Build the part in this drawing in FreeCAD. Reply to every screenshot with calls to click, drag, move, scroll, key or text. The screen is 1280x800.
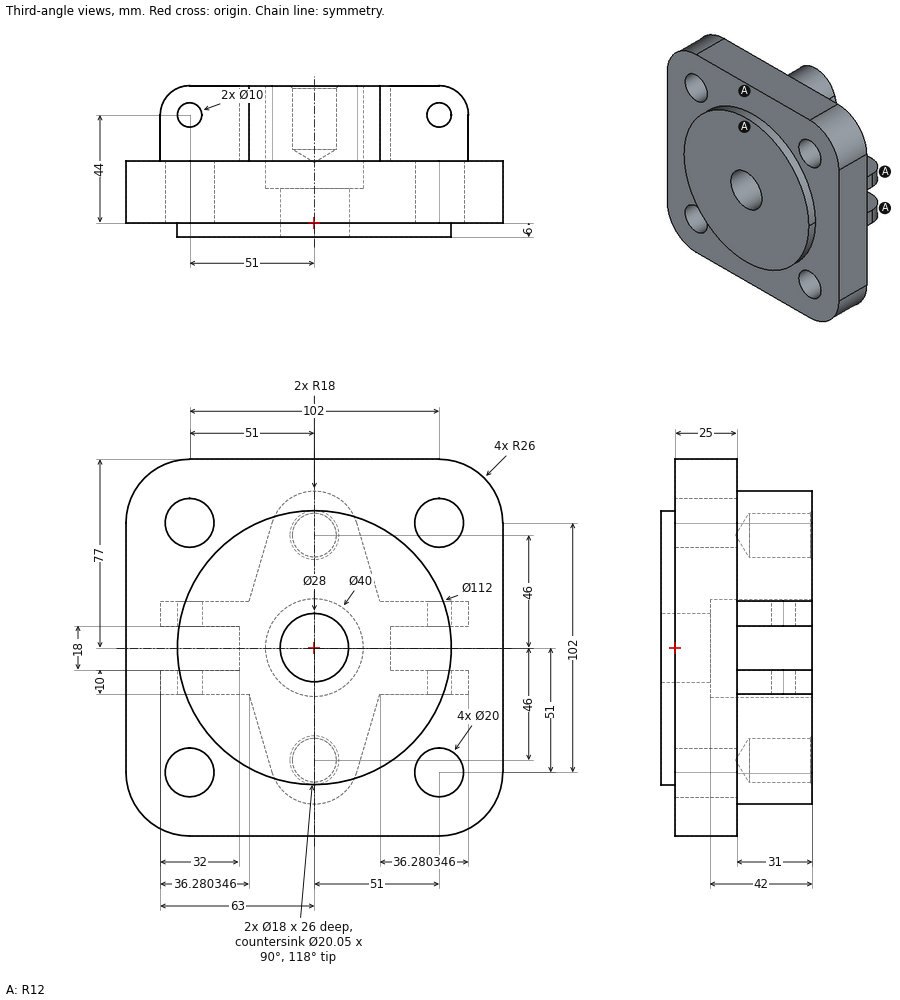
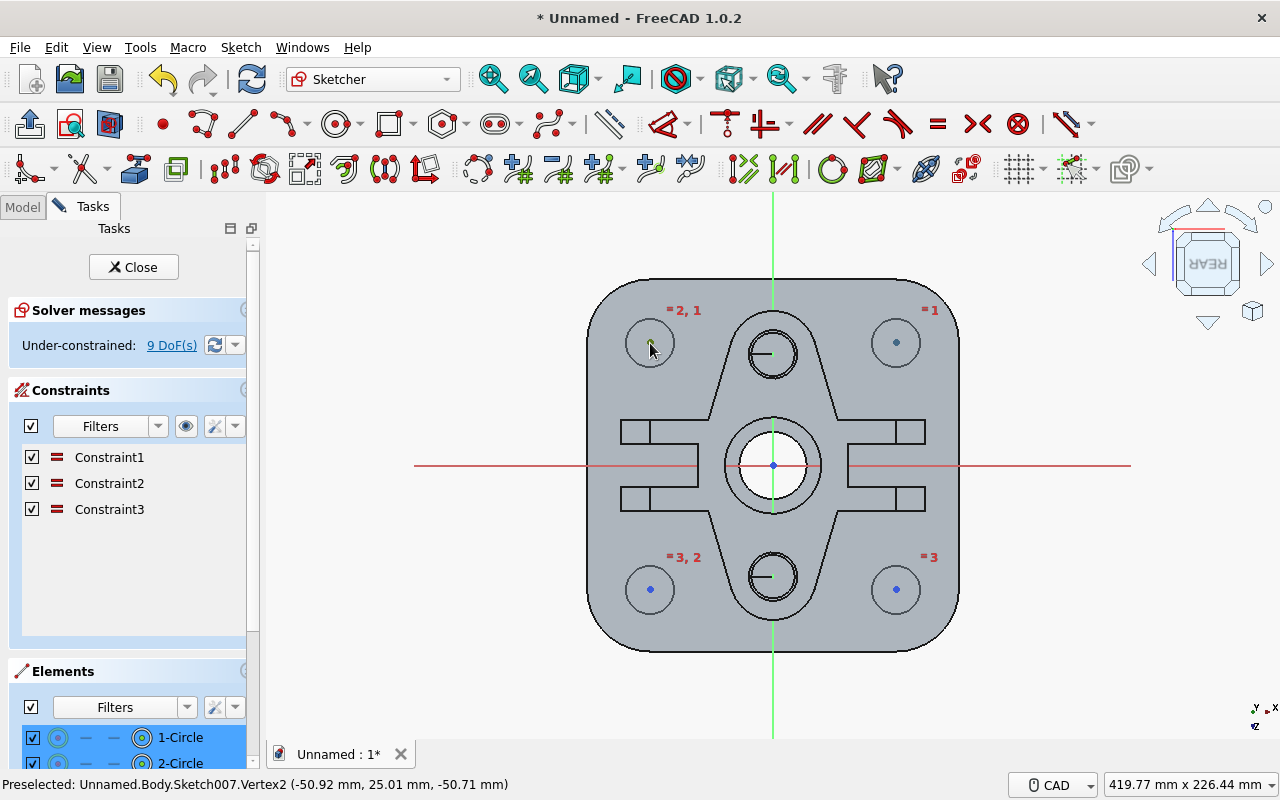
click(773, 676)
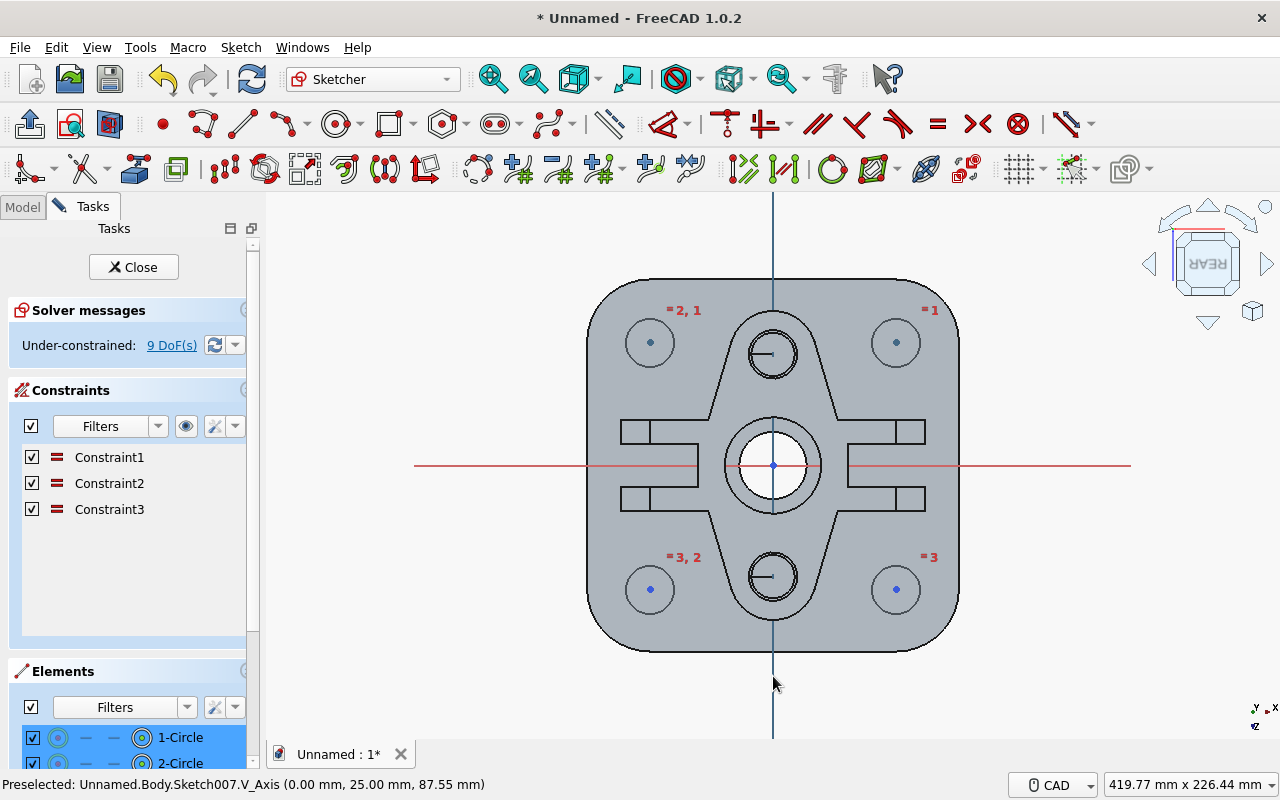
key(s)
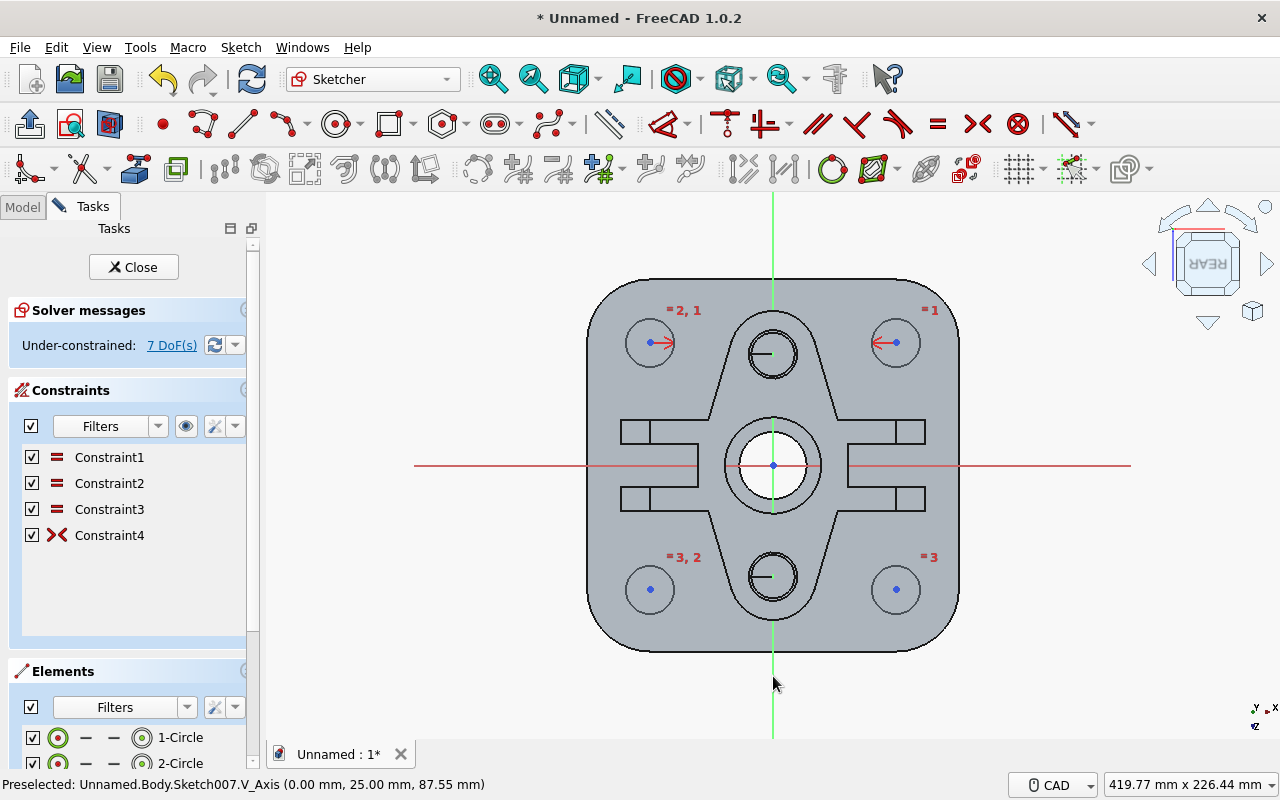
click(650, 343)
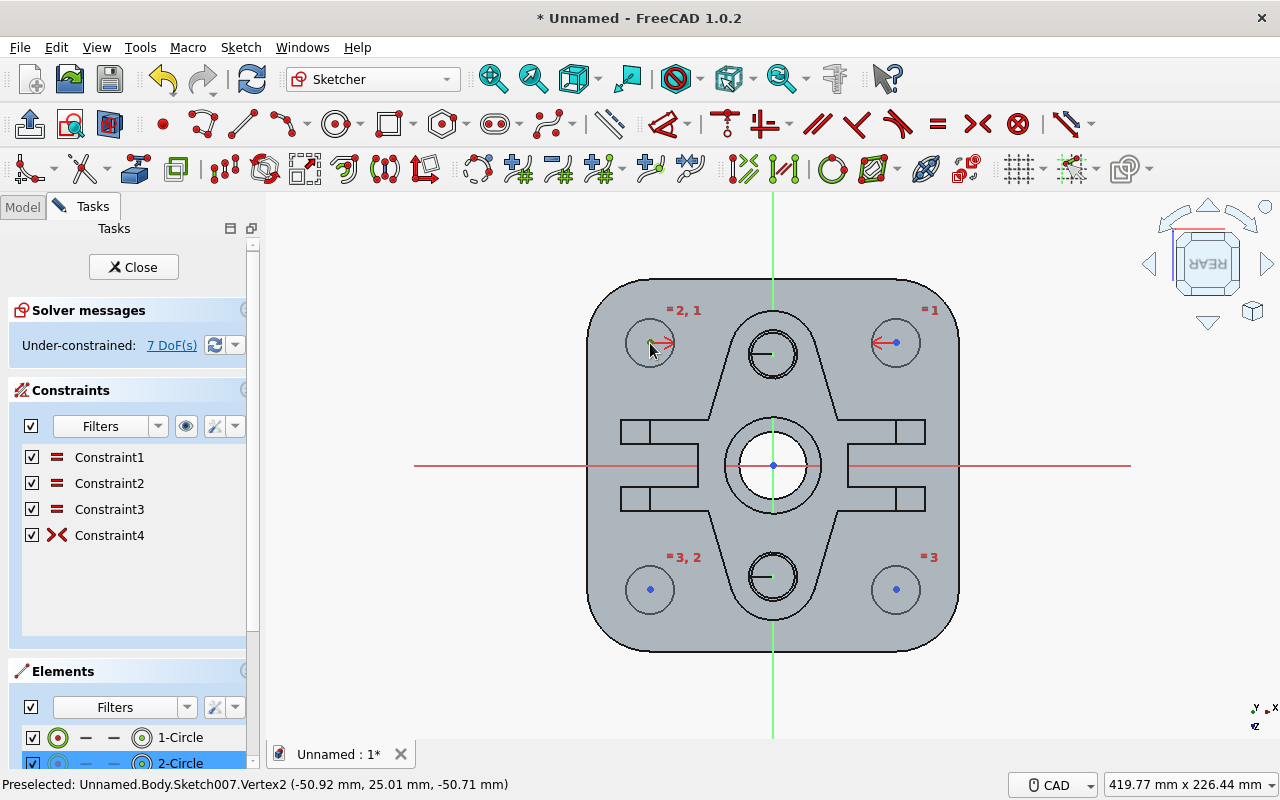
click(650, 590)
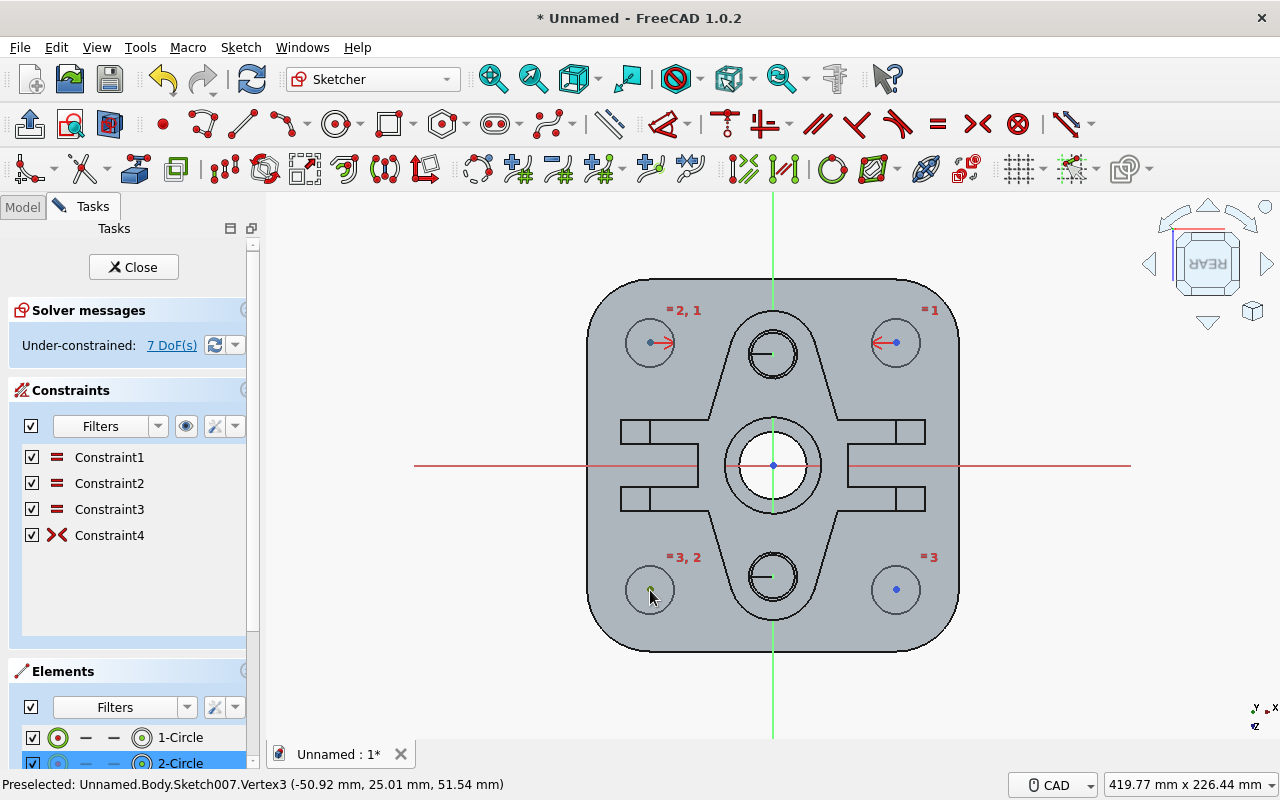
click(411, 465)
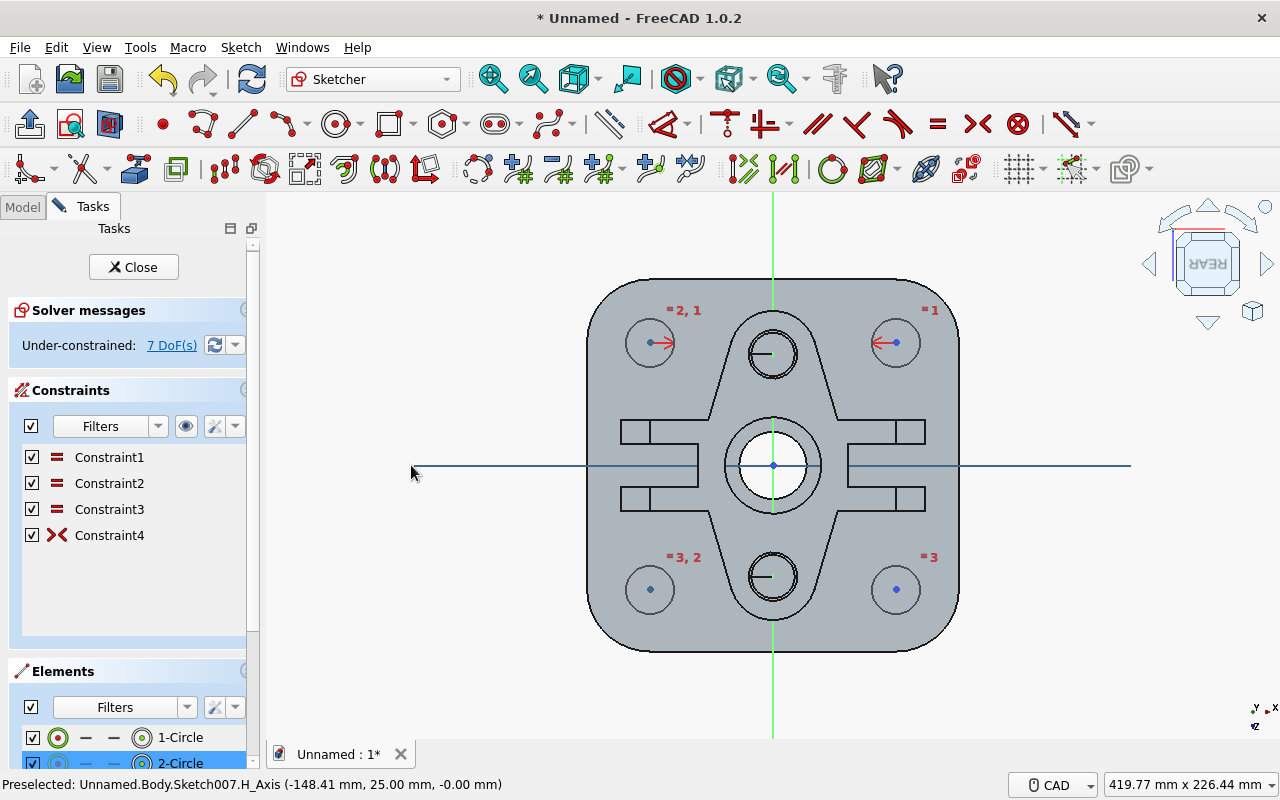
key(s)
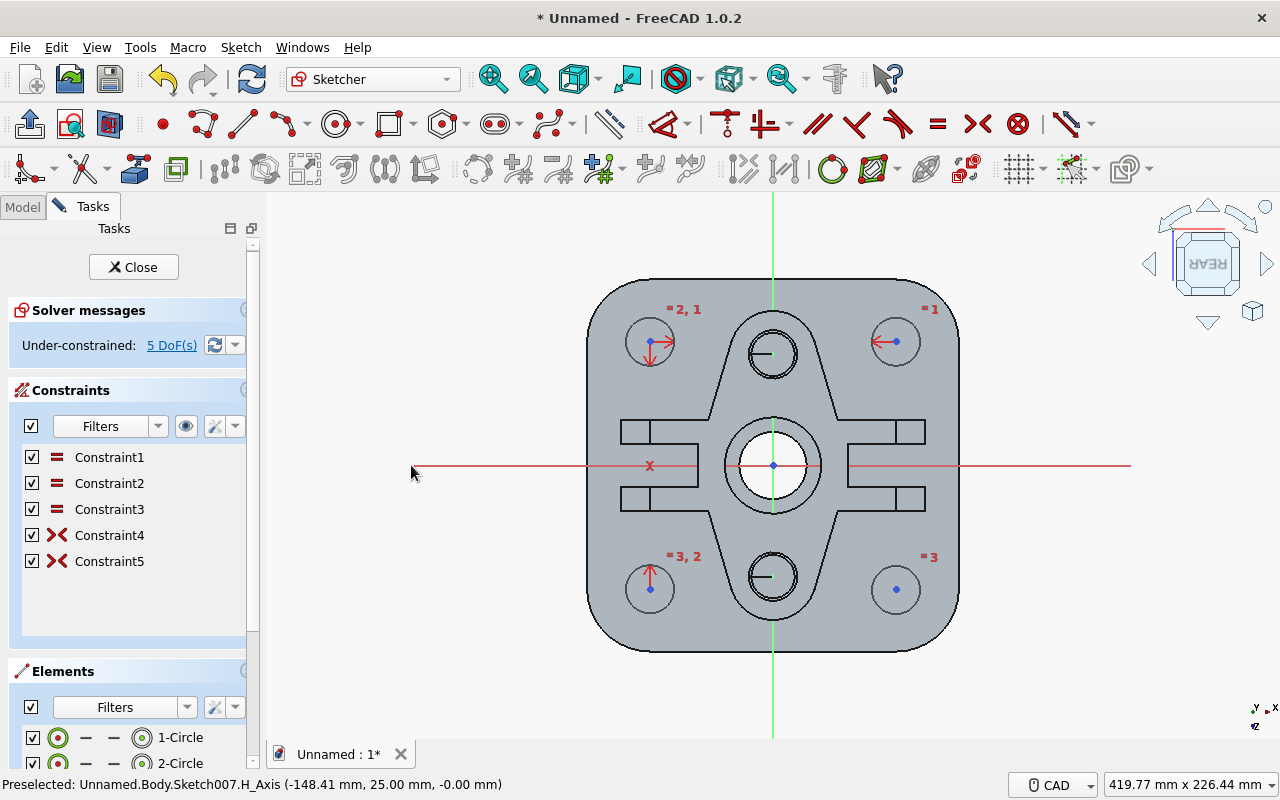
click(896, 342)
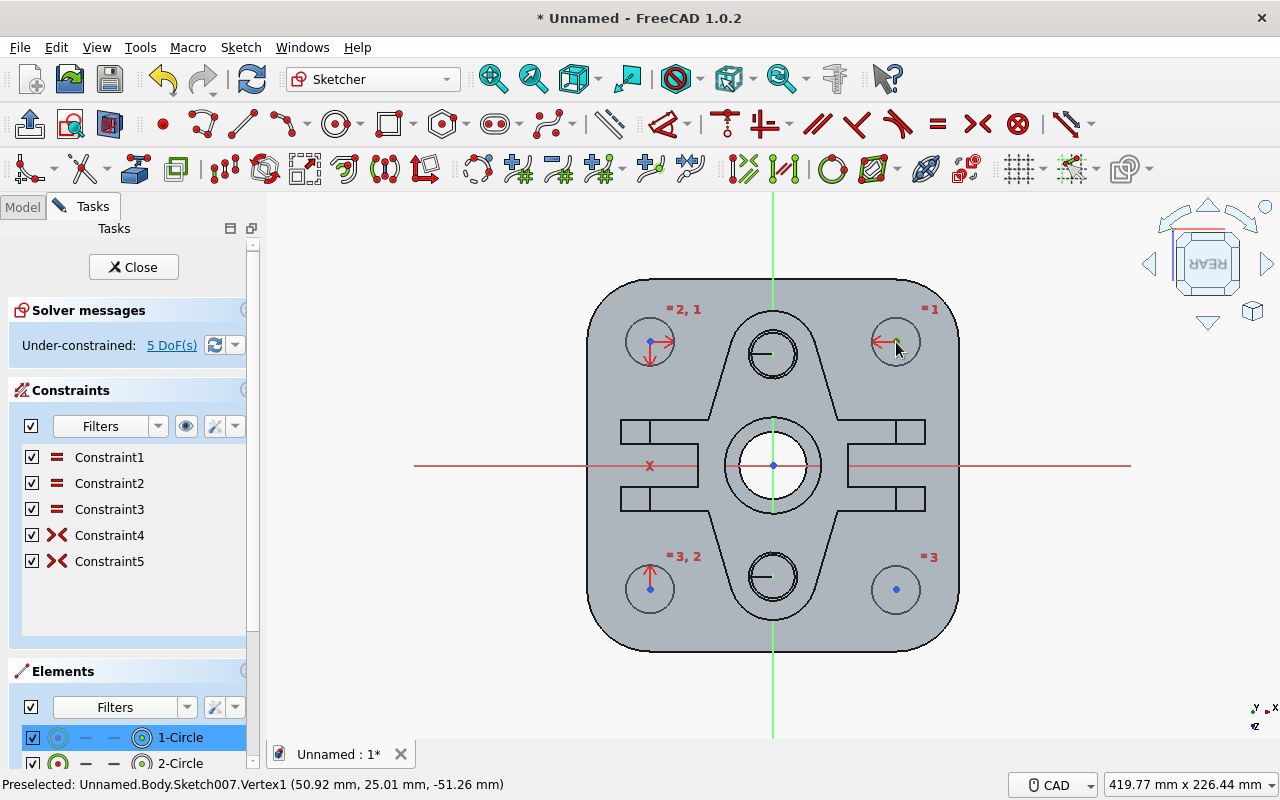
click(896, 590)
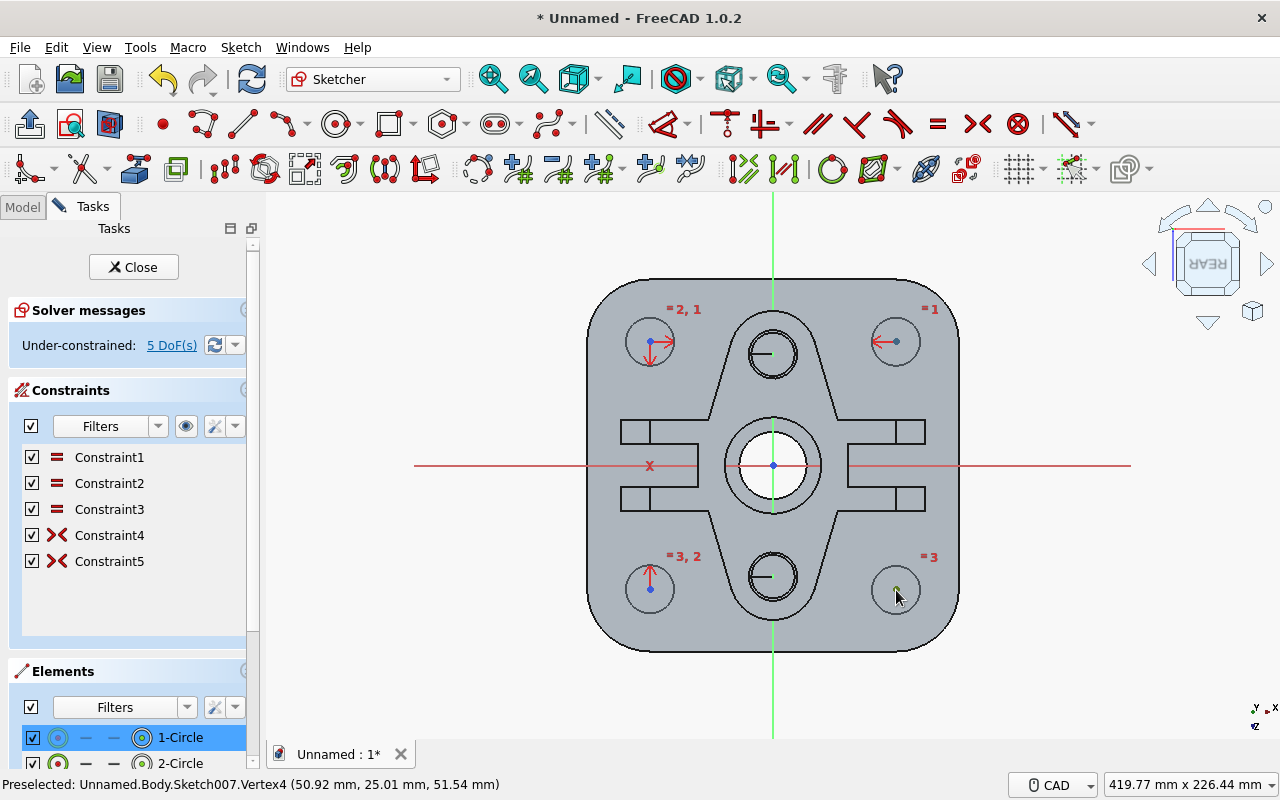
click(411, 465)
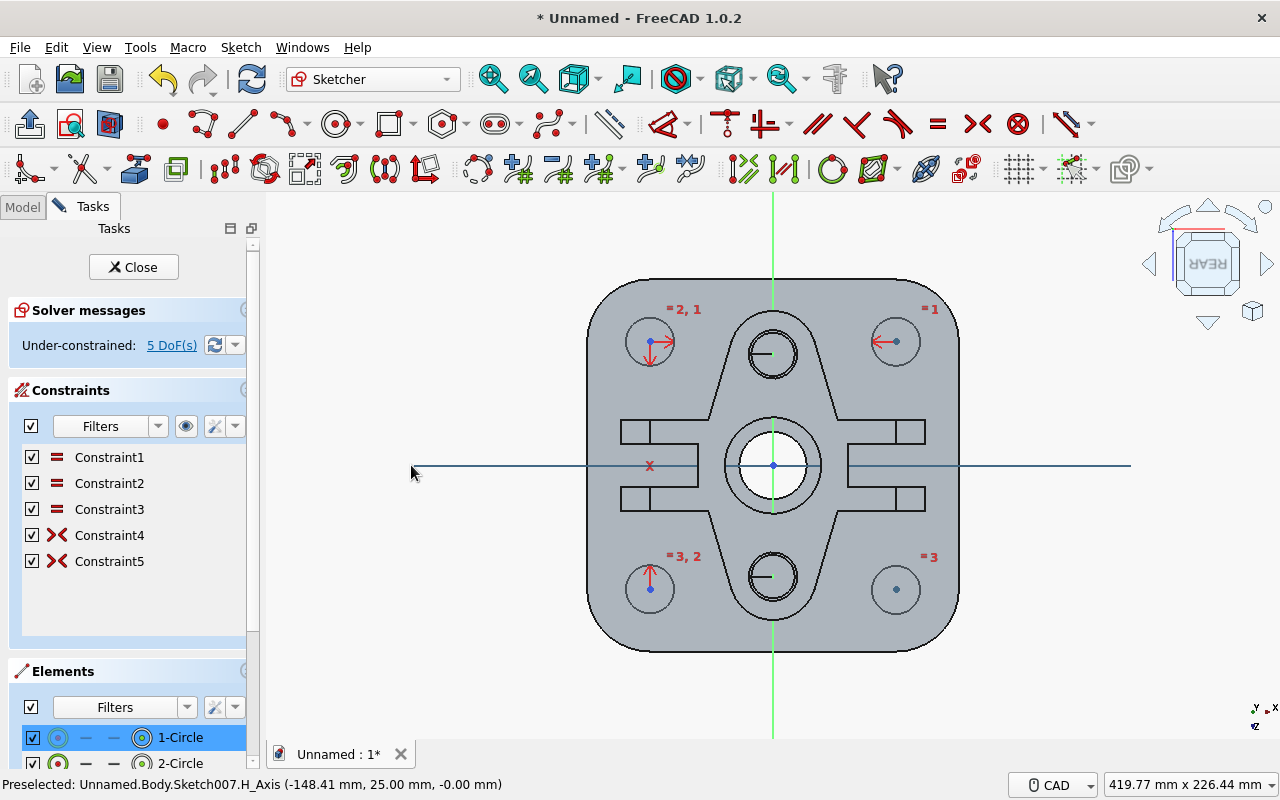
key(s)